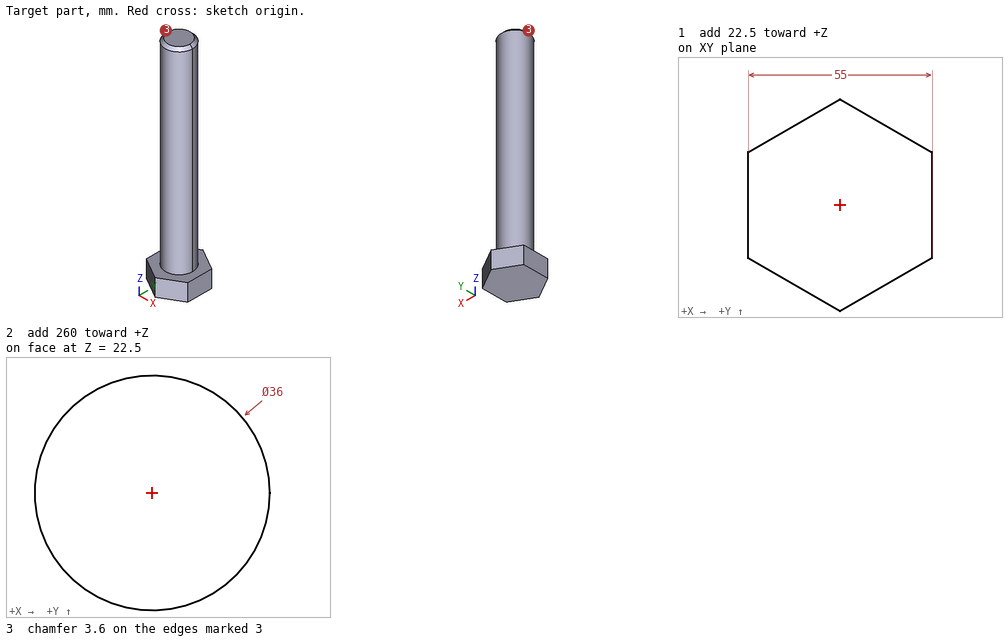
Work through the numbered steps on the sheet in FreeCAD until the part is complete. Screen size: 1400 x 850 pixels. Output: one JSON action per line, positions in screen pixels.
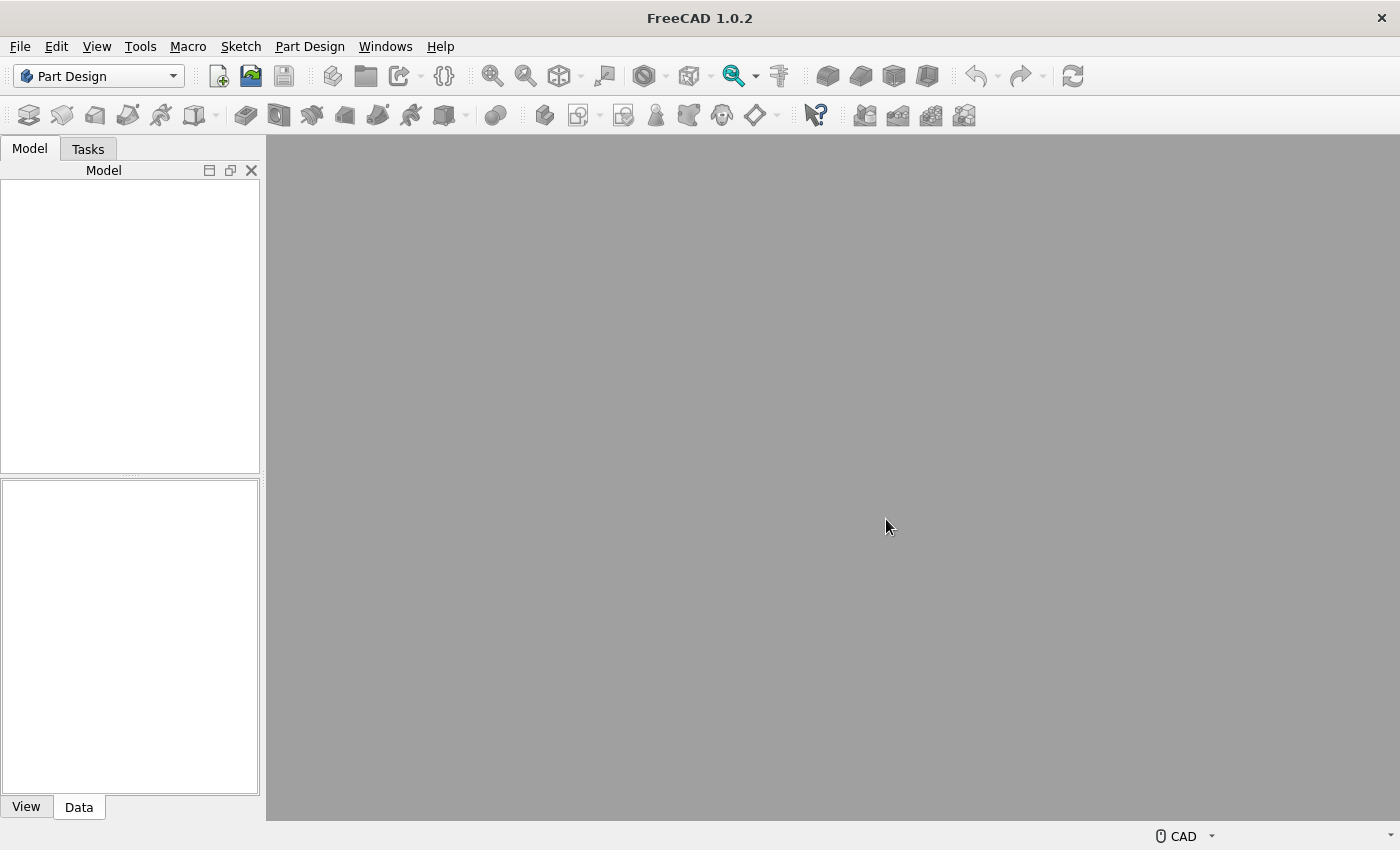
{"action": "left_click", "coordinate": [218, 76]}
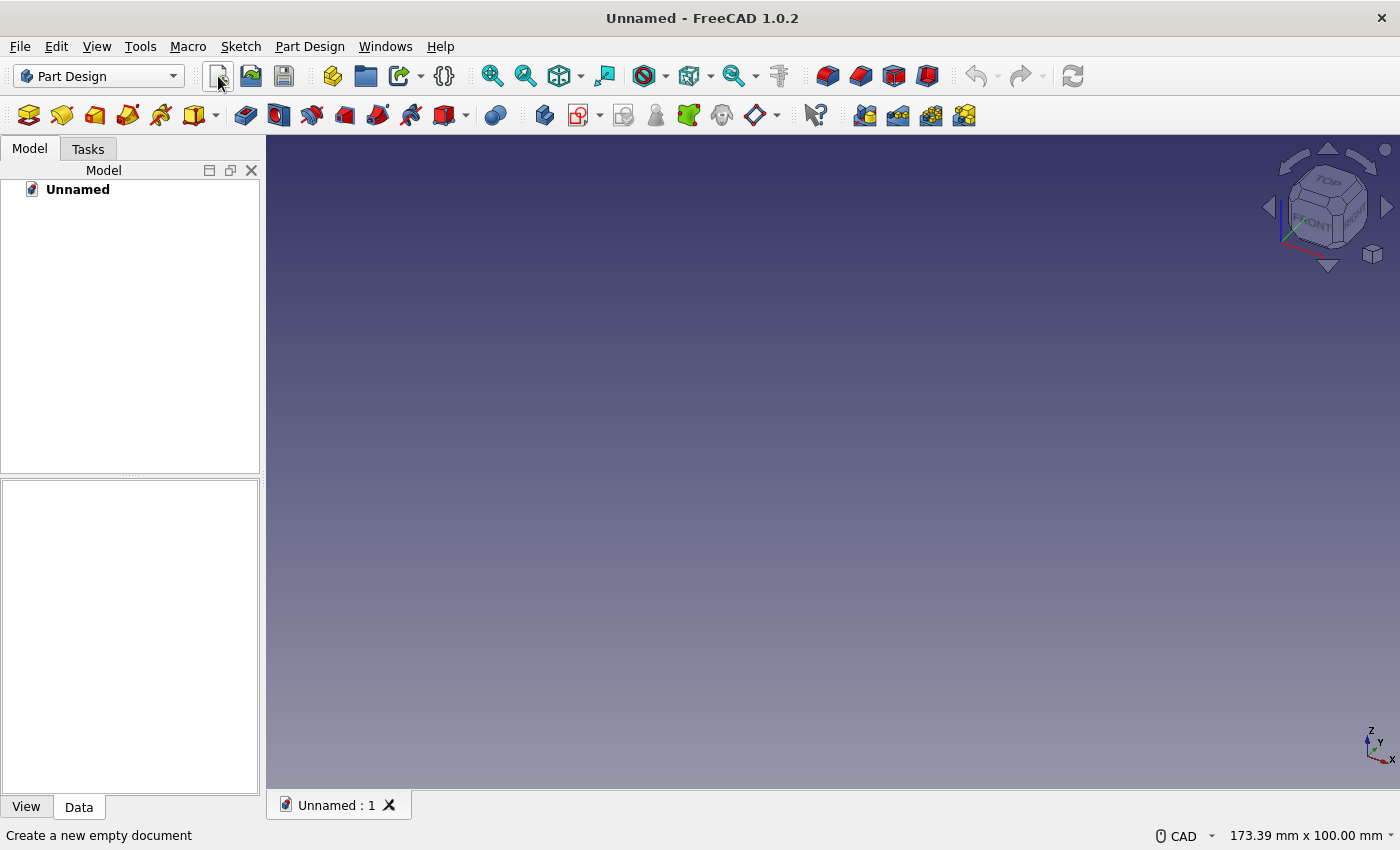
{"action": "left_click", "coordinate": [578, 116]}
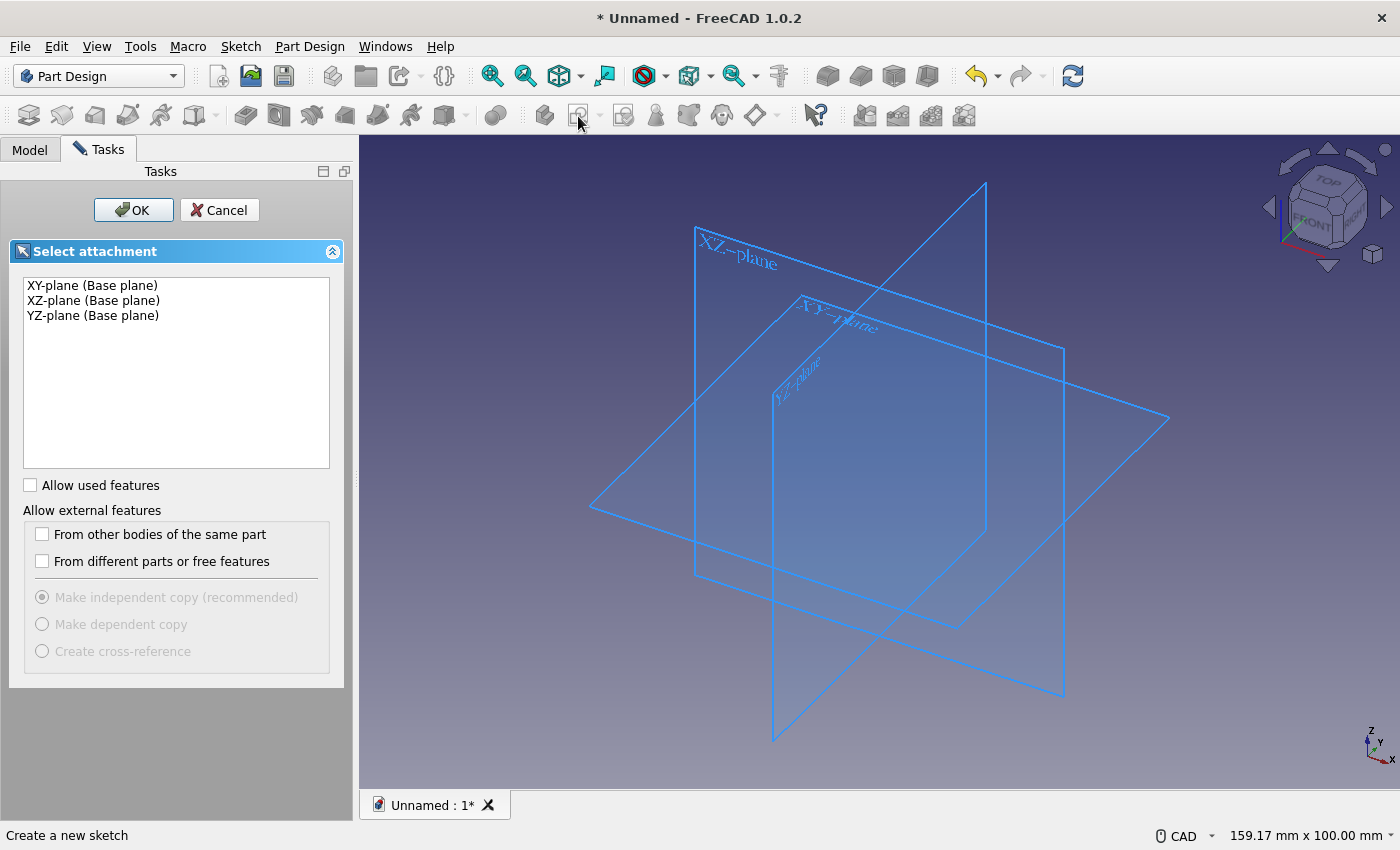
{"action": "left_click", "coordinate": [84, 286]}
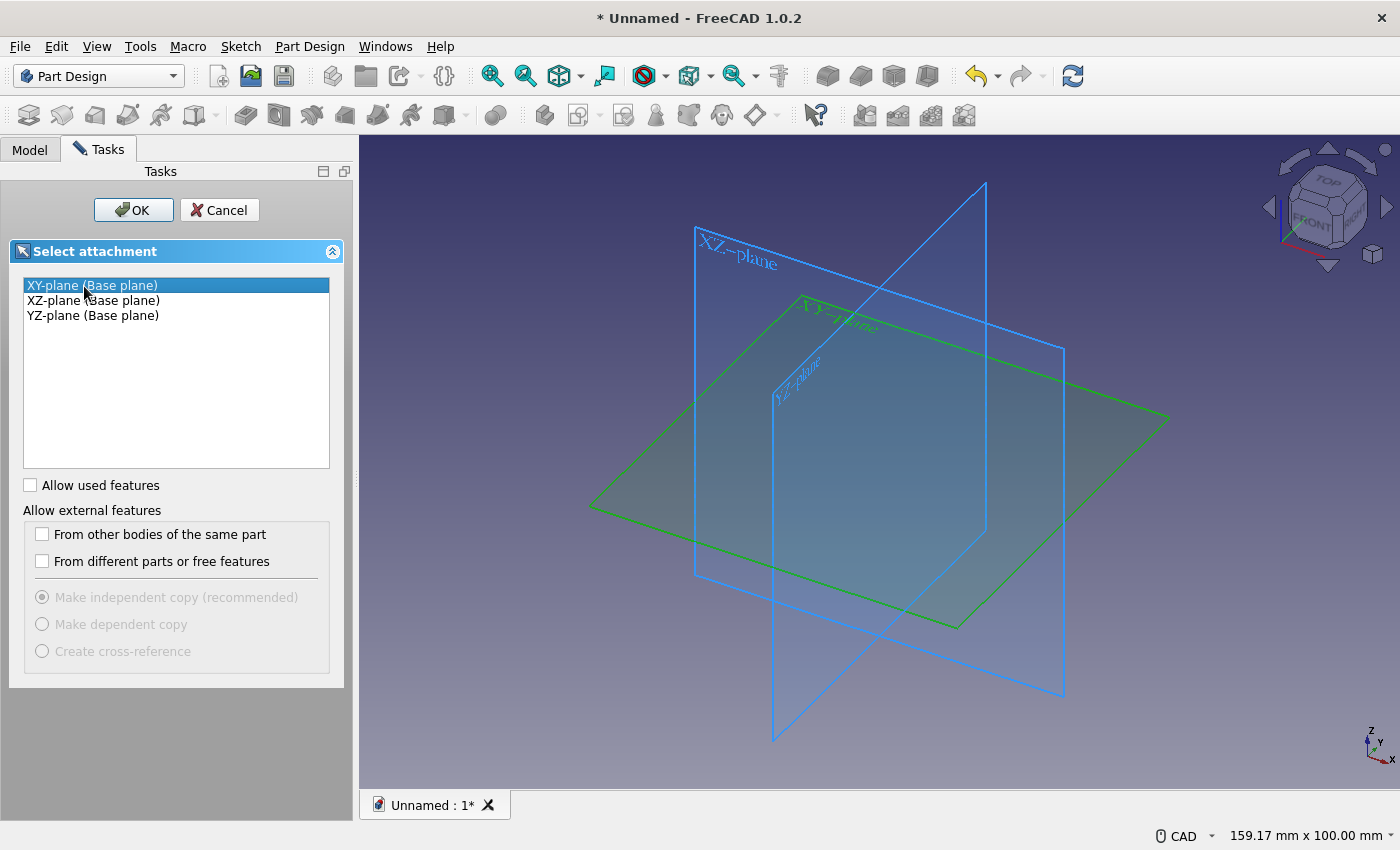
{"action": "left_click", "coordinate": [134, 210]}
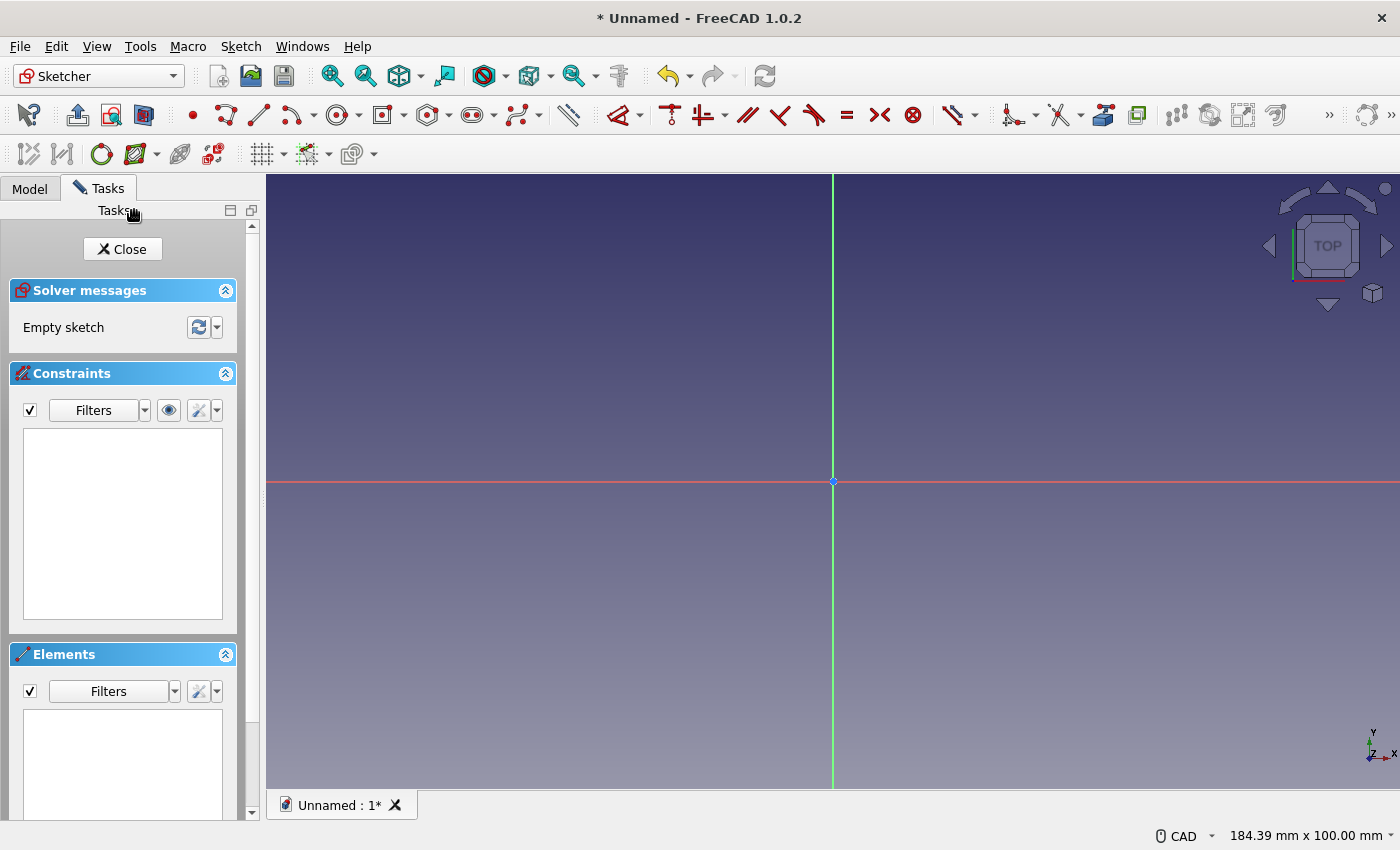
{"action": "left_click", "coordinate": [426, 116]}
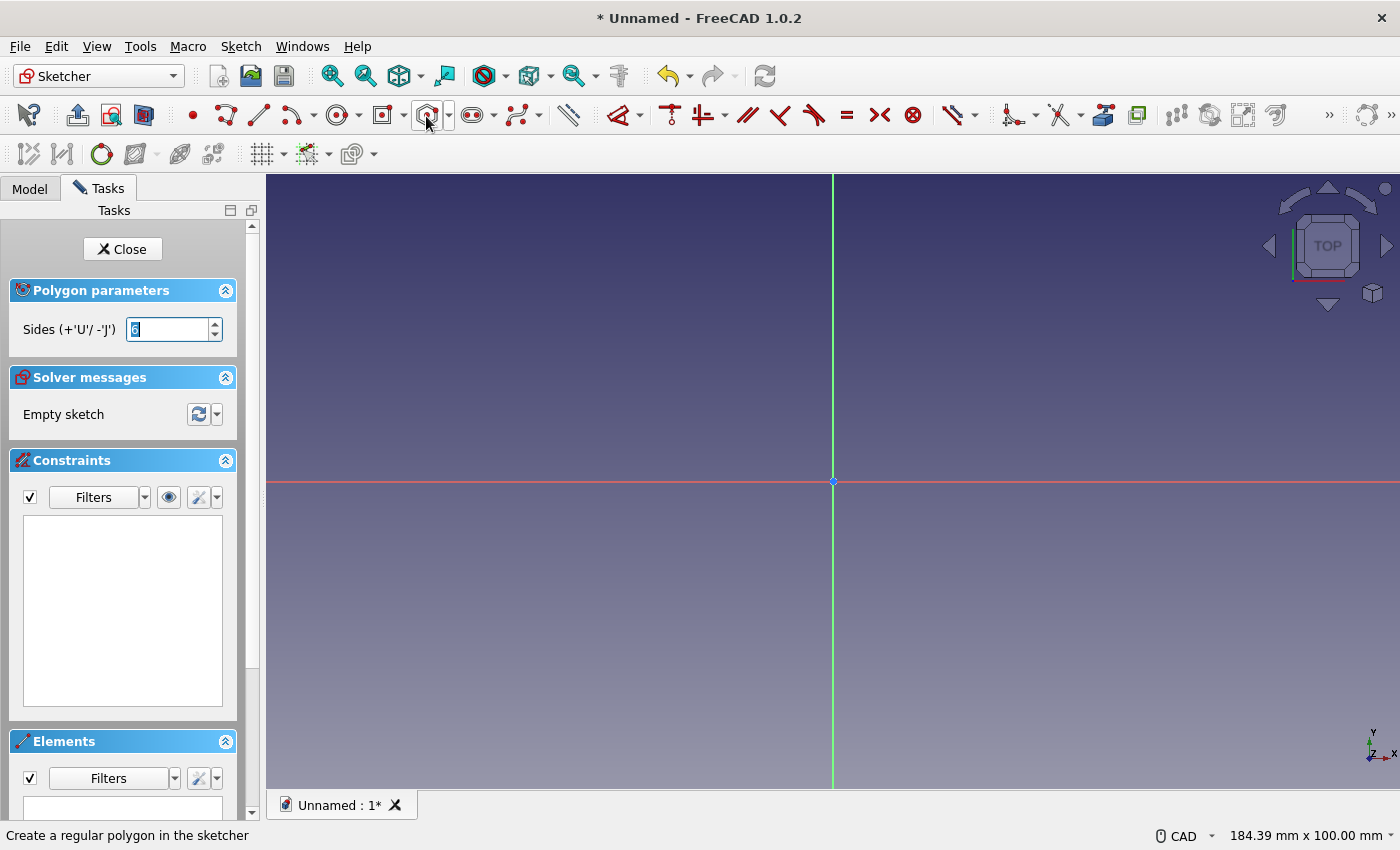
{"action": "left_click", "coordinate": [833, 482]}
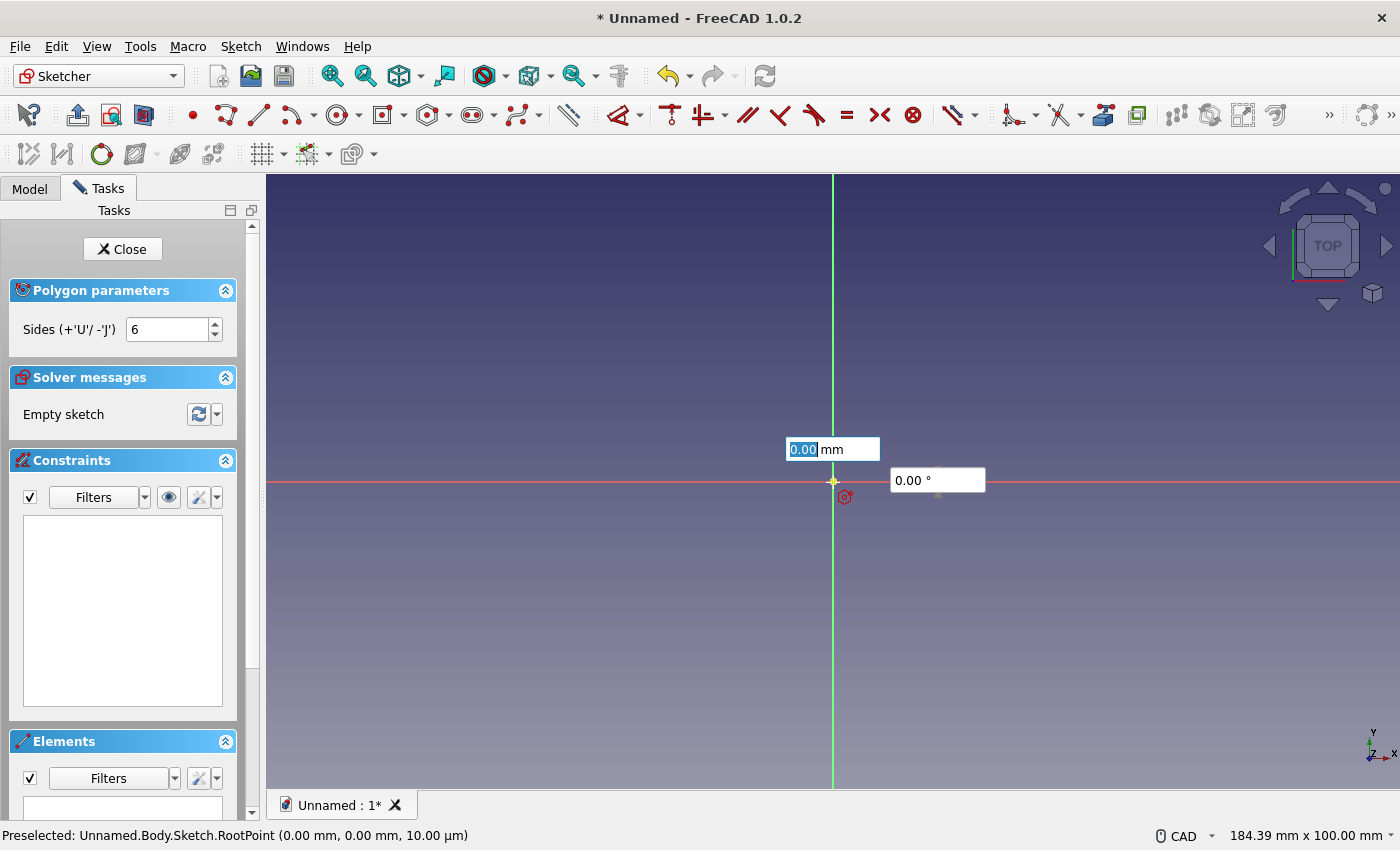
{"action": "left_click", "coordinate": [833, 286]}
{"action": "right_click", "coordinate": [833, 286]}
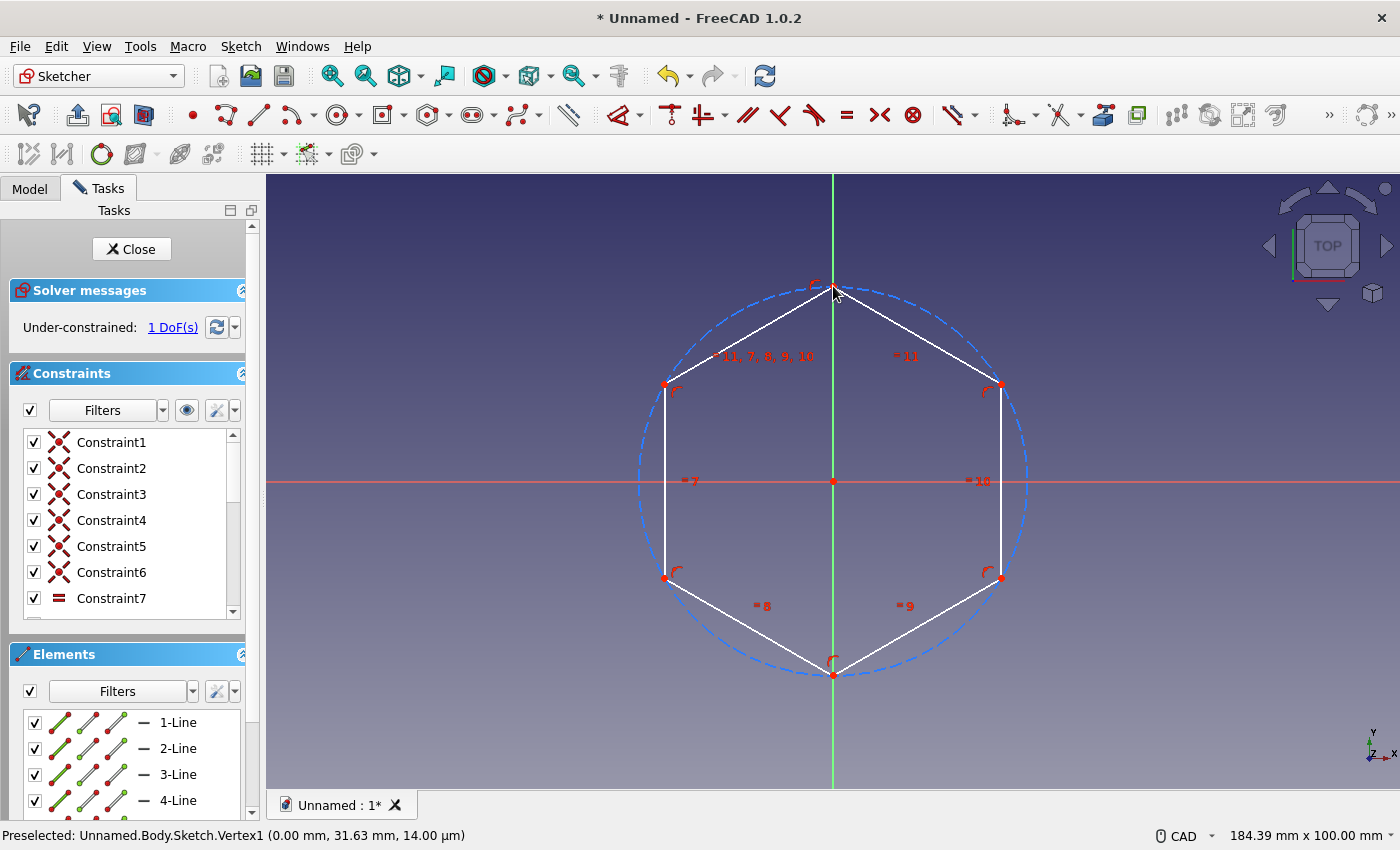
{"action": "left_click", "coordinate": [665, 384]}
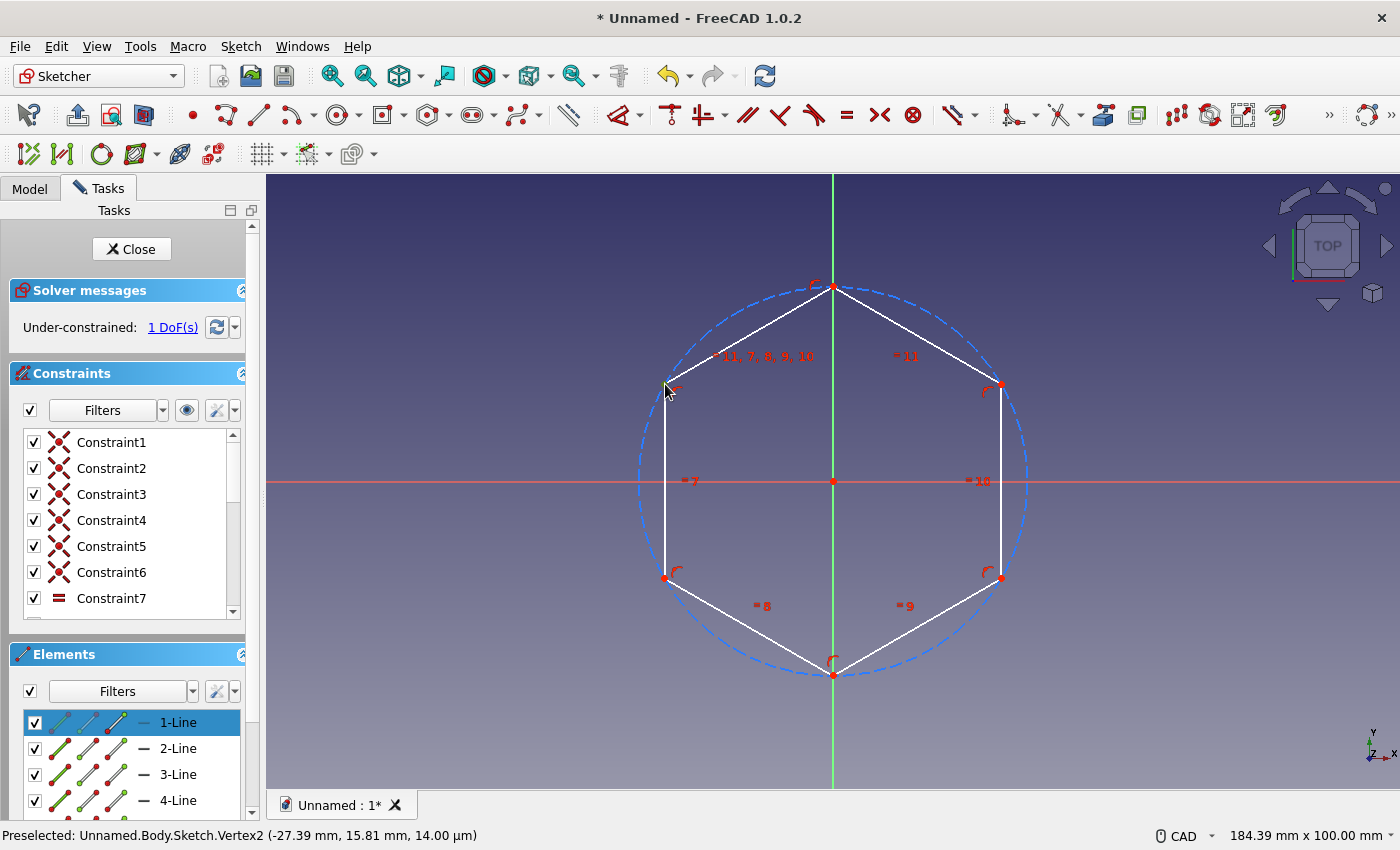
{"action": "left_click", "coordinate": [1001, 579]}